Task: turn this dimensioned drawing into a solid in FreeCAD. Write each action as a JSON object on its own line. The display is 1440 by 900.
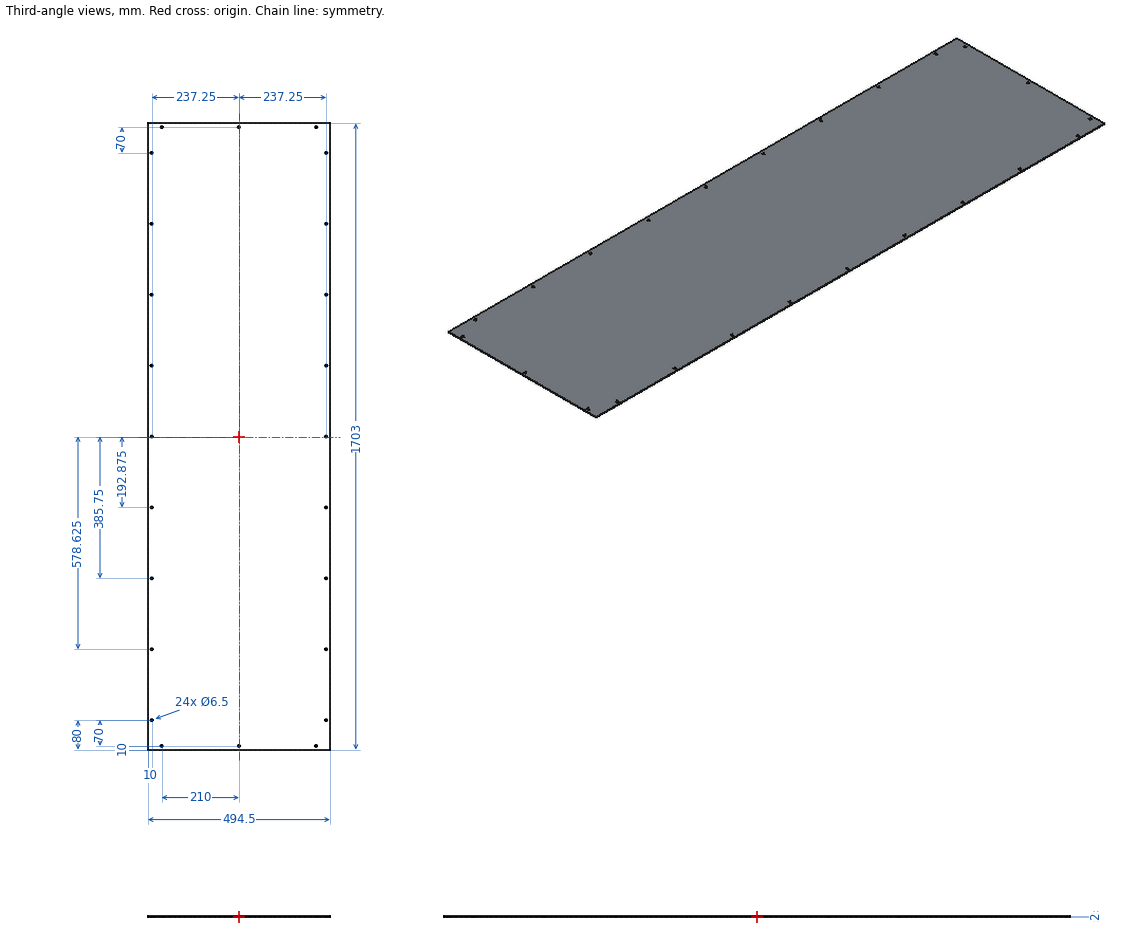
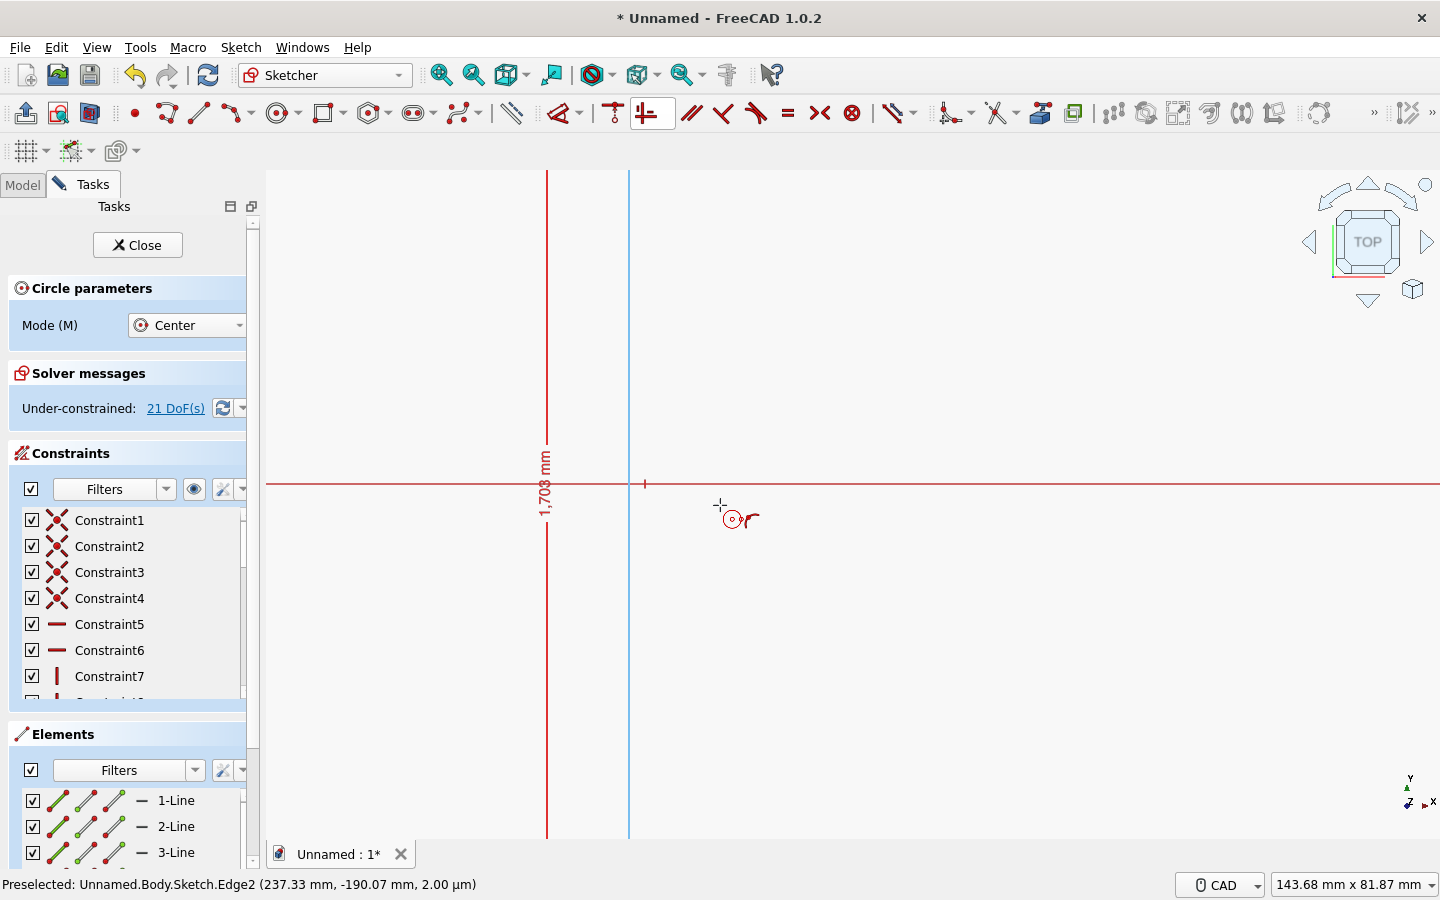
{"action": "scroll", "coordinate": [720, 505], "scroll_direction": "down", "scroll_amount": 17}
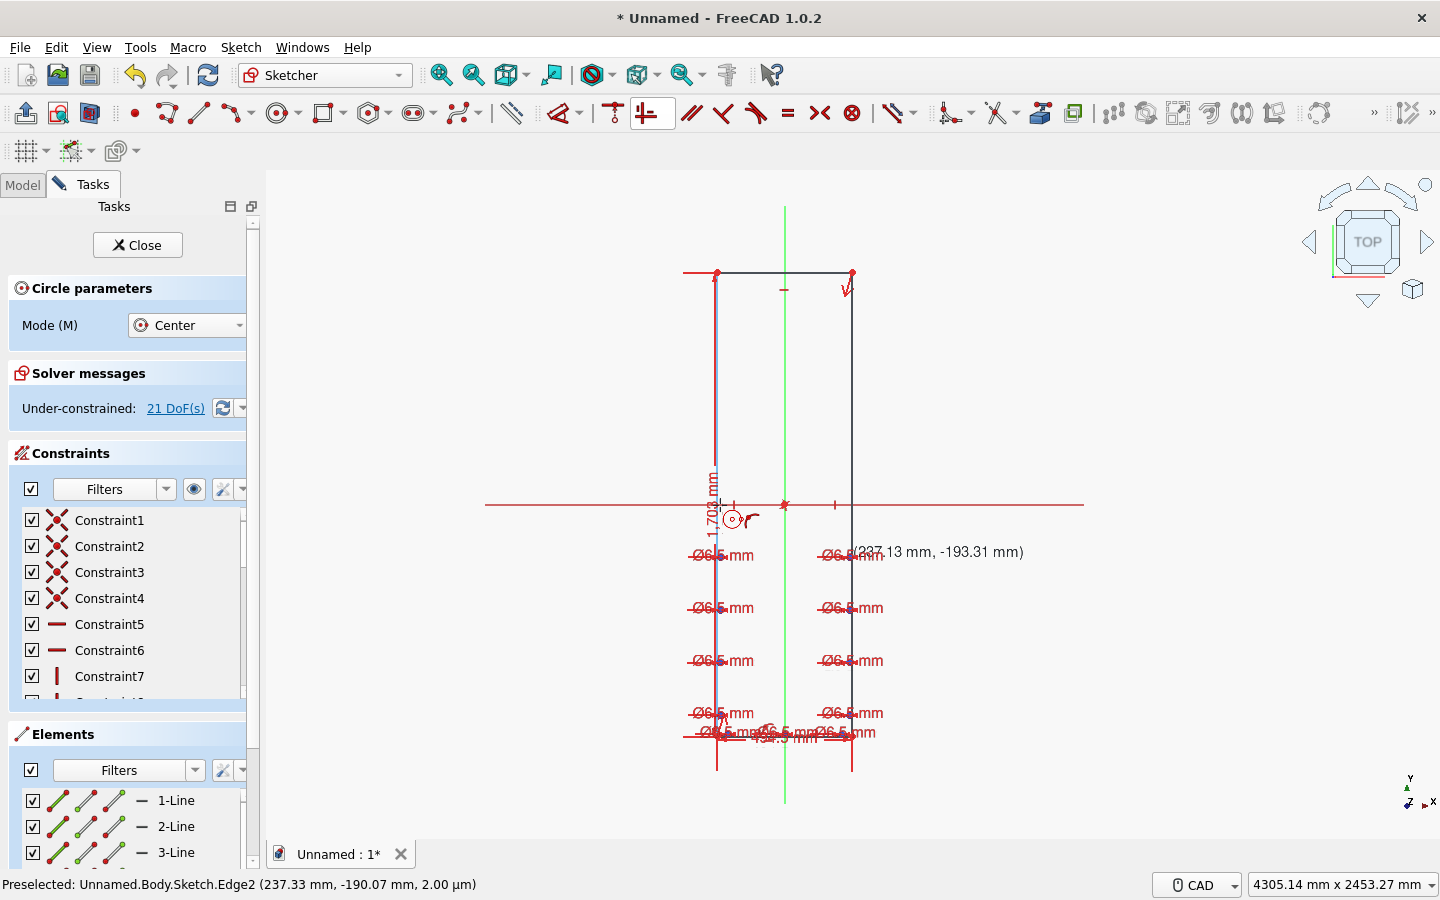
{"action": "scroll", "coordinate": [720, 505], "scroll_direction": "up", "scroll_amount": 9}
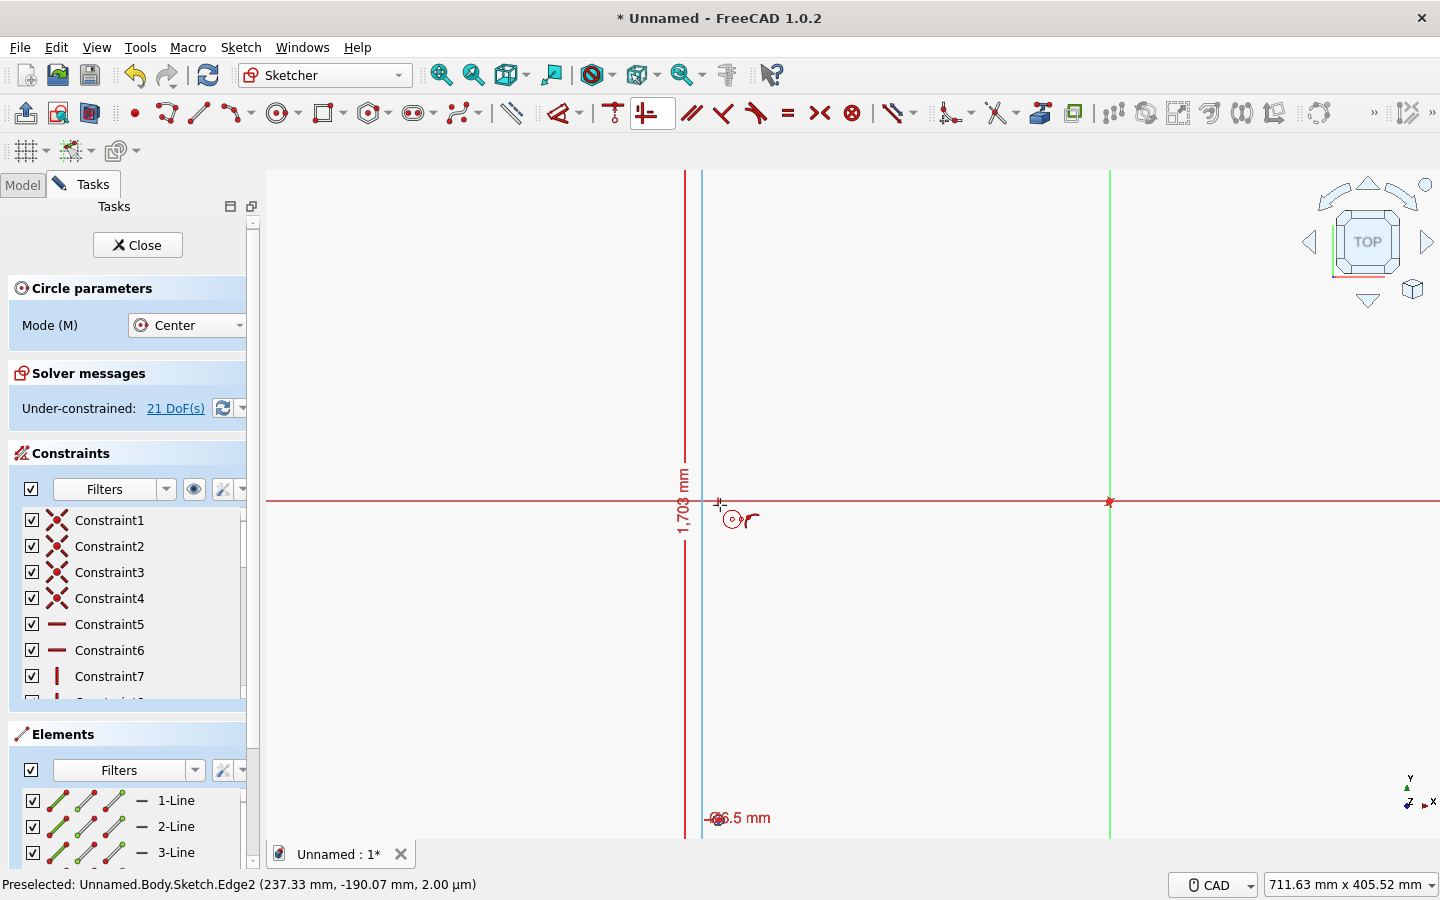
{"action": "left_click", "coordinate": [718, 501]}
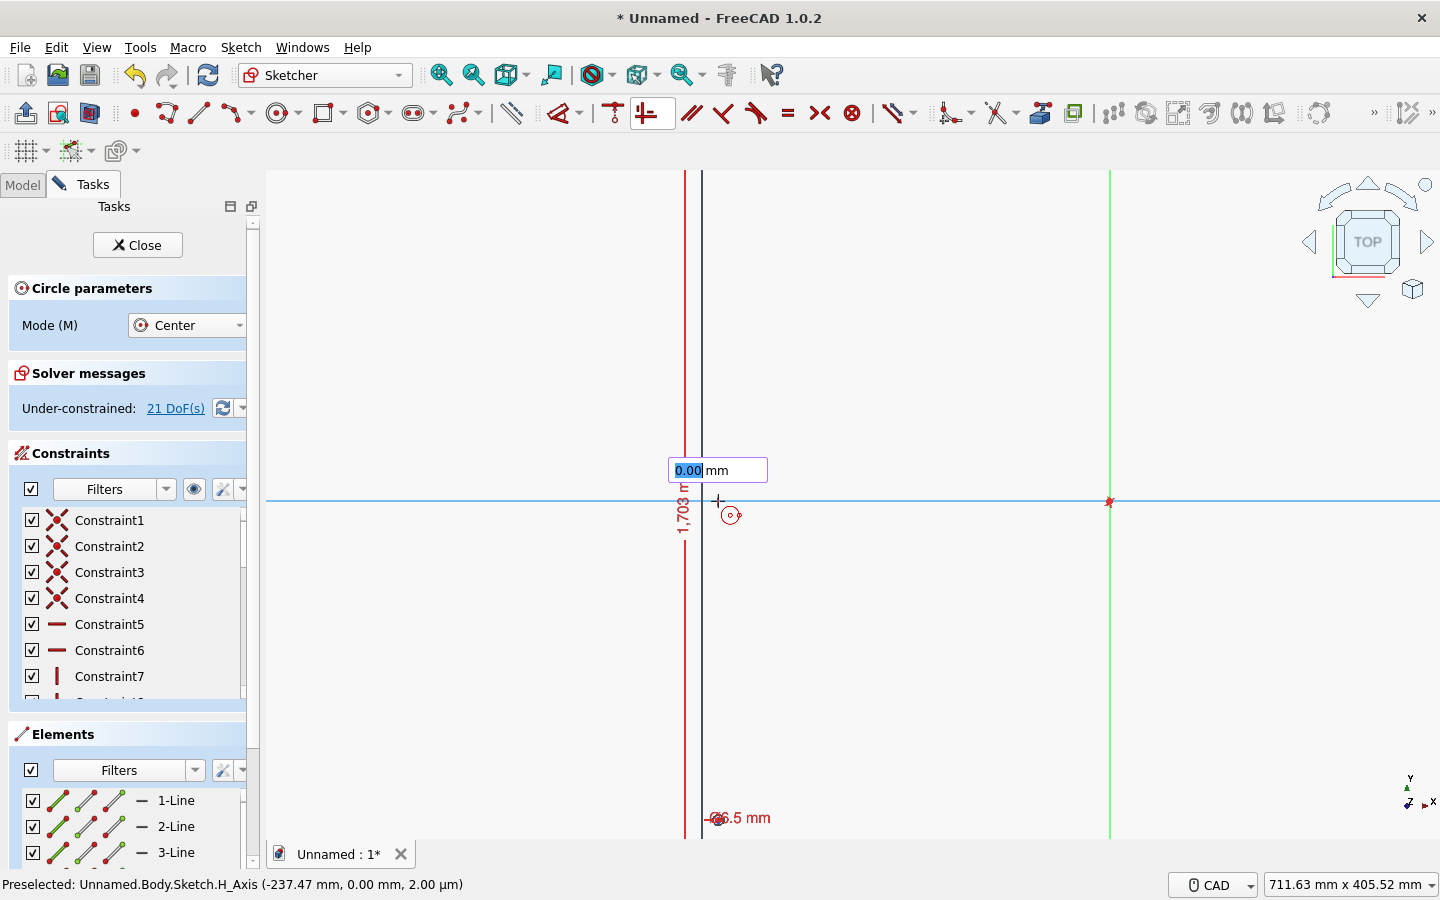
{"action": "scroll", "coordinate": [720, 496], "scroll_direction": "up", "scroll_amount": 6}
{"action": "mouse_move", "coordinate": [720, 495]}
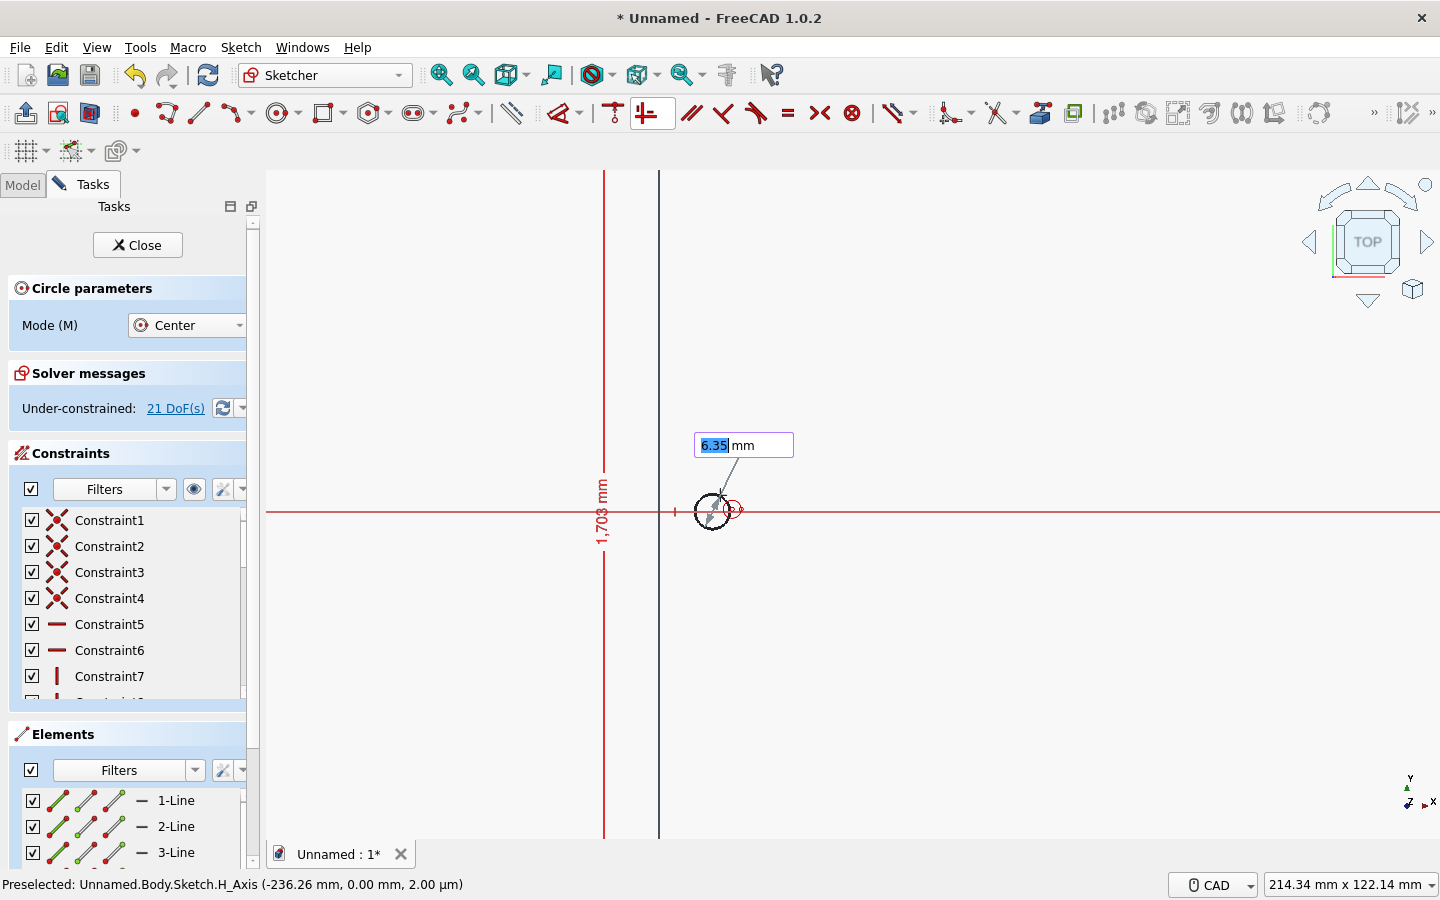
{"action": "type", "text": "6.5"}
{"action": "key", "text": "Return"}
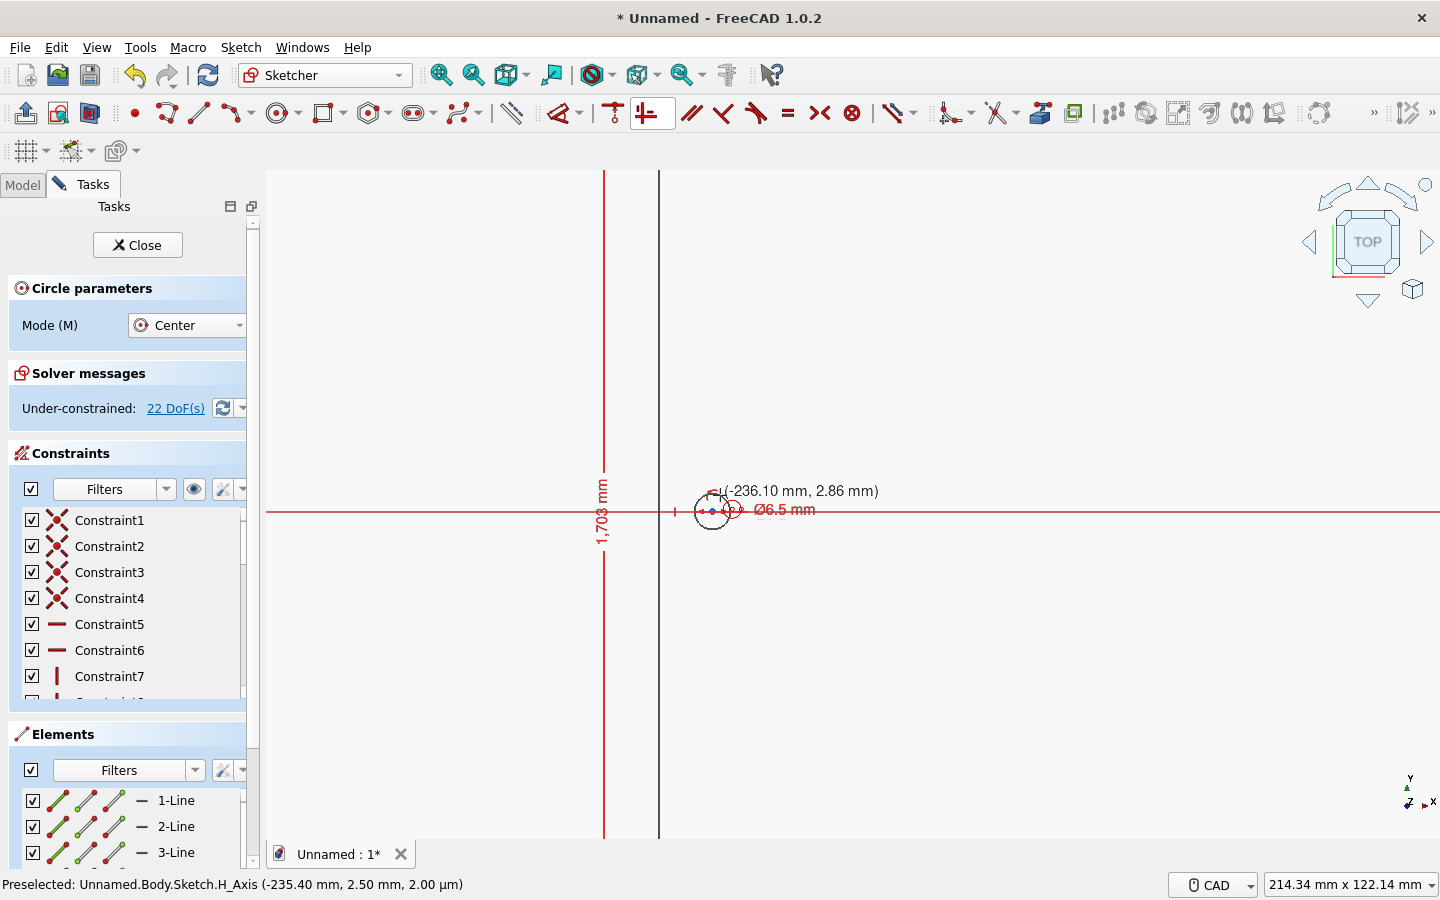
{"action": "scroll", "coordinate": [720, 504], "scroll_direction": "down", "scroll_amount": 15}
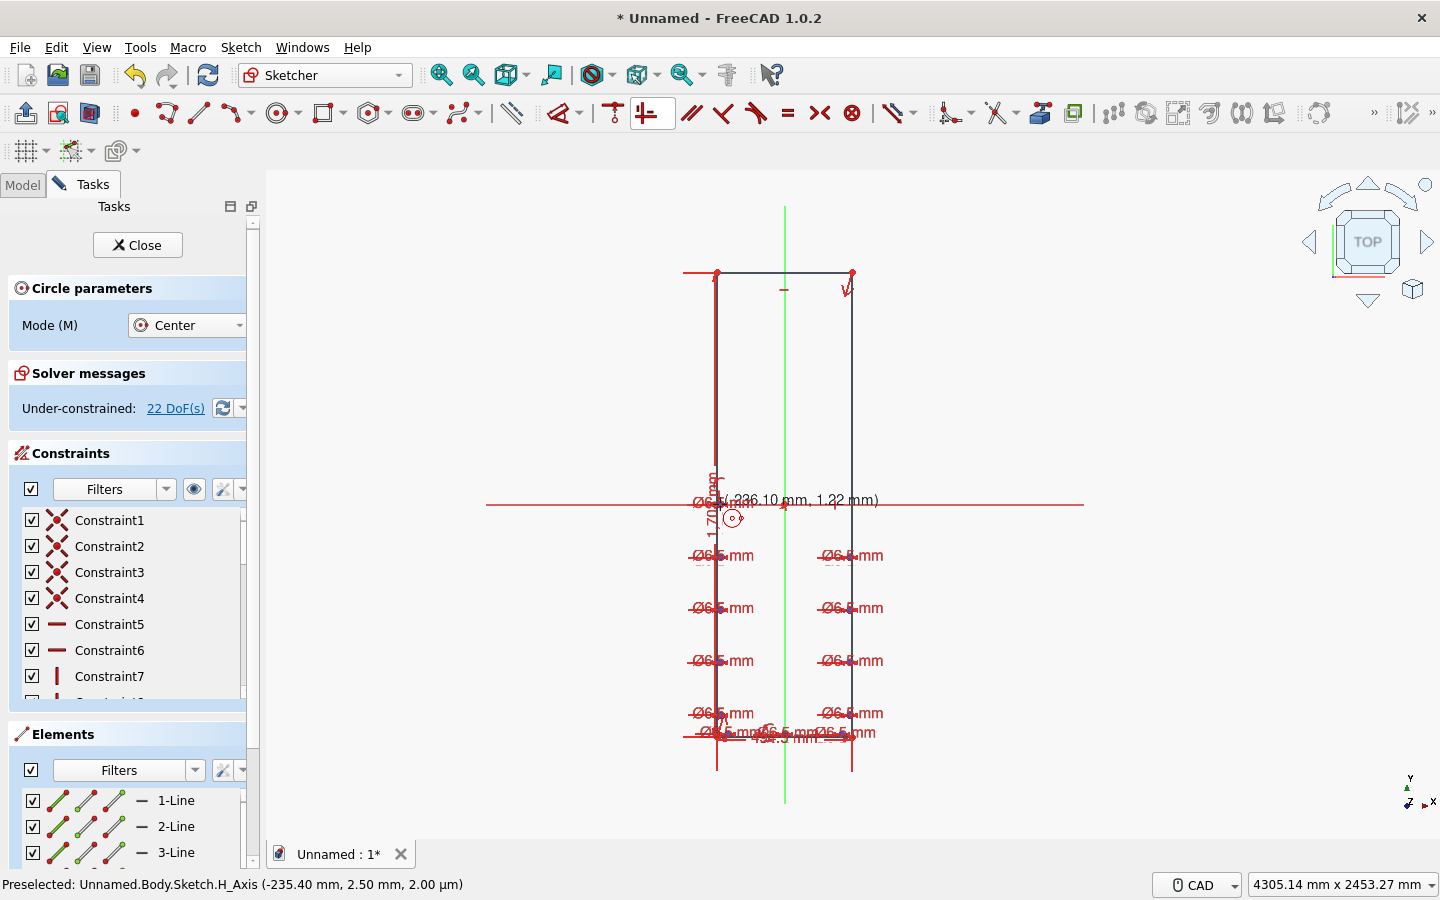
{"action": "scroll", "coordinate": [720, 452], "scroll_direction": "up", "scroll_amount": 17}